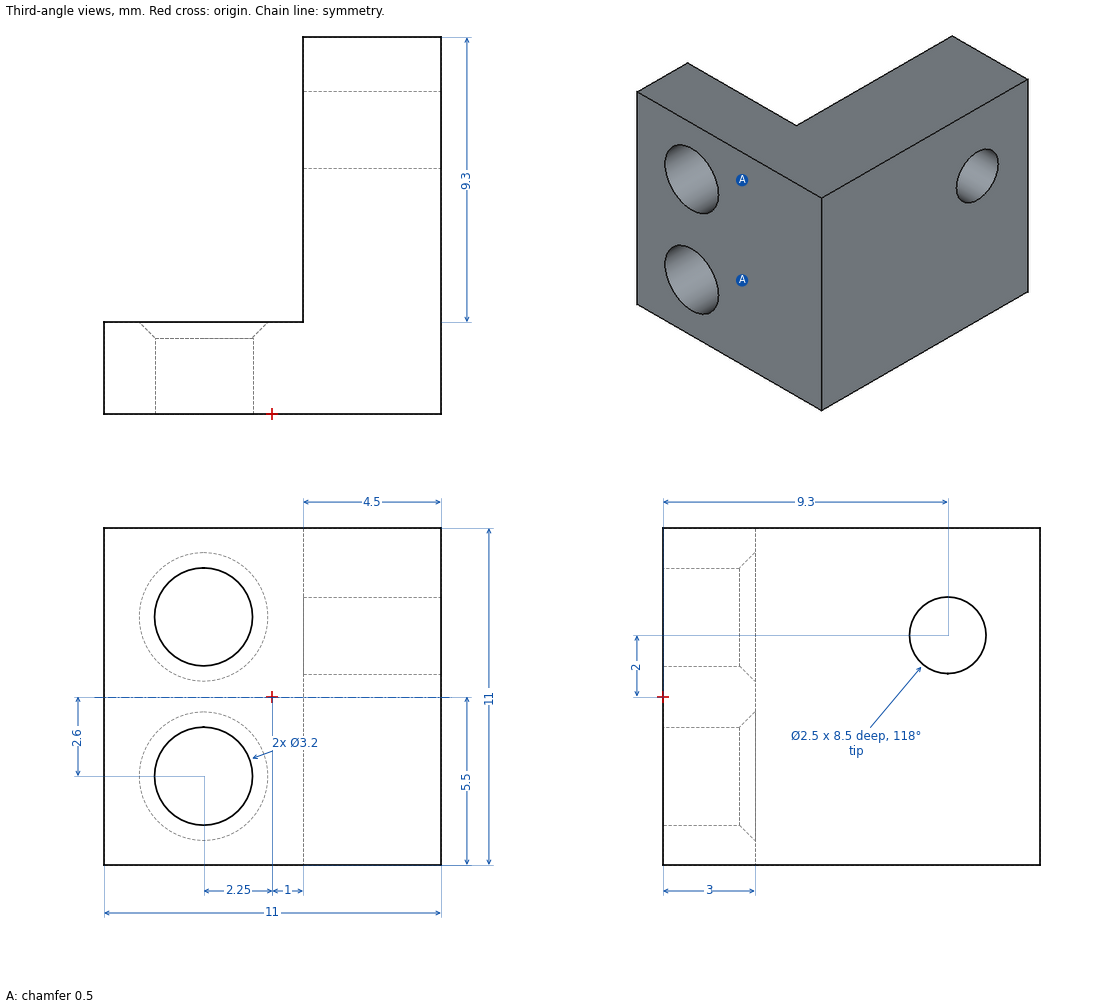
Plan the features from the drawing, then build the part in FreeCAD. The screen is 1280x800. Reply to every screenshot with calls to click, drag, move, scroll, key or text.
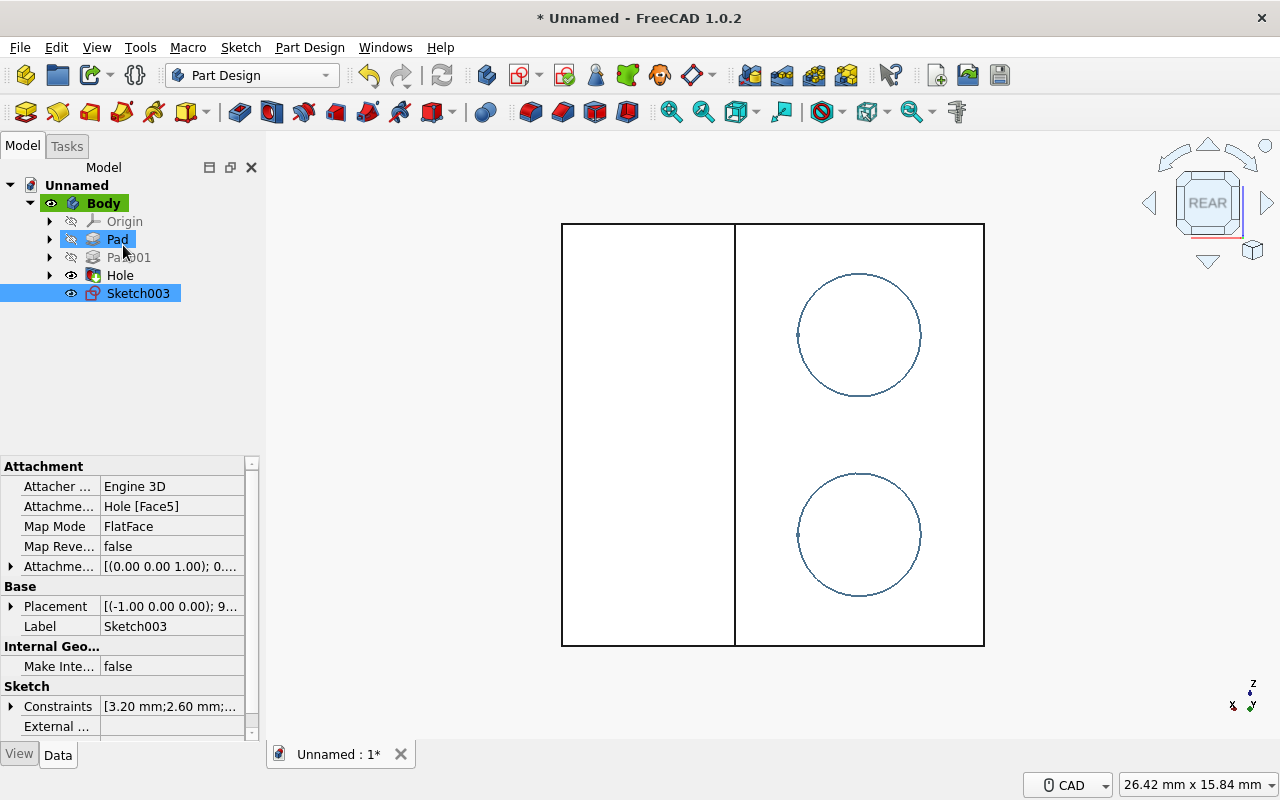
click(240, 112)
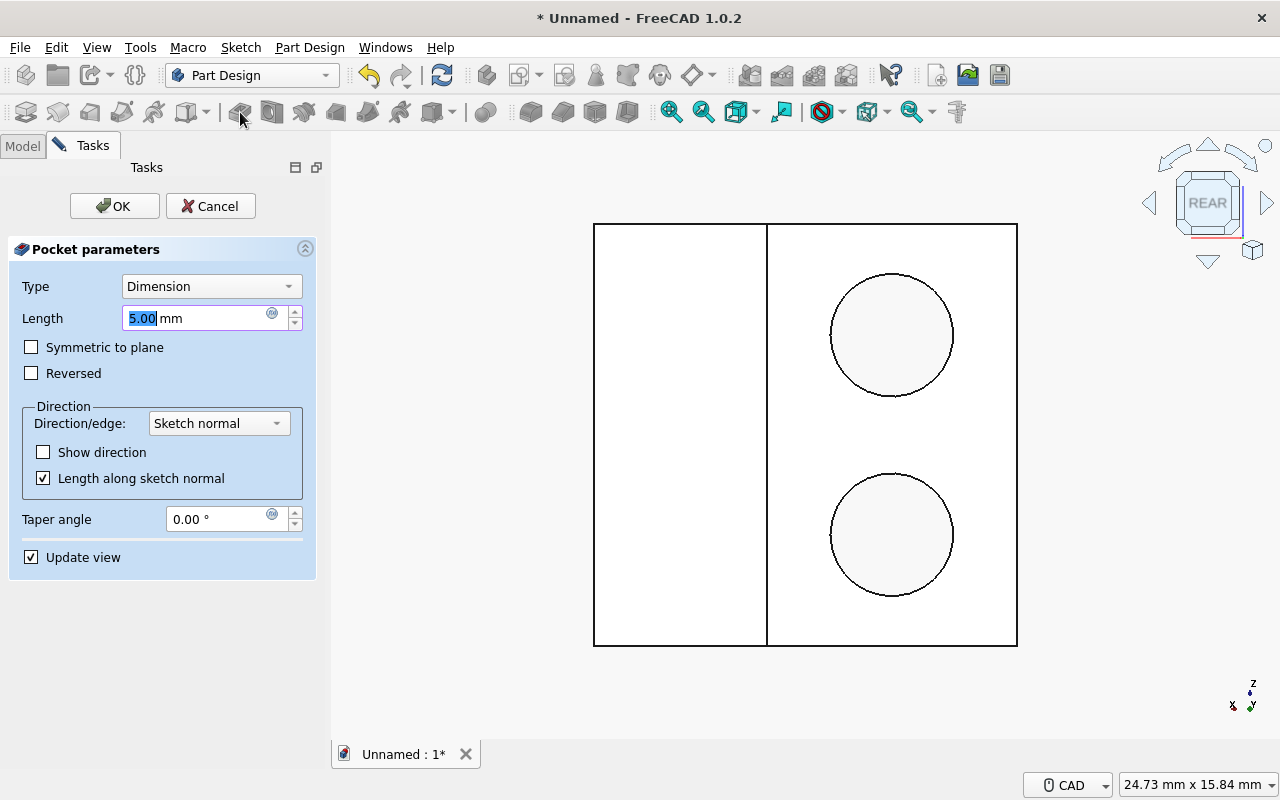
click(212, 286)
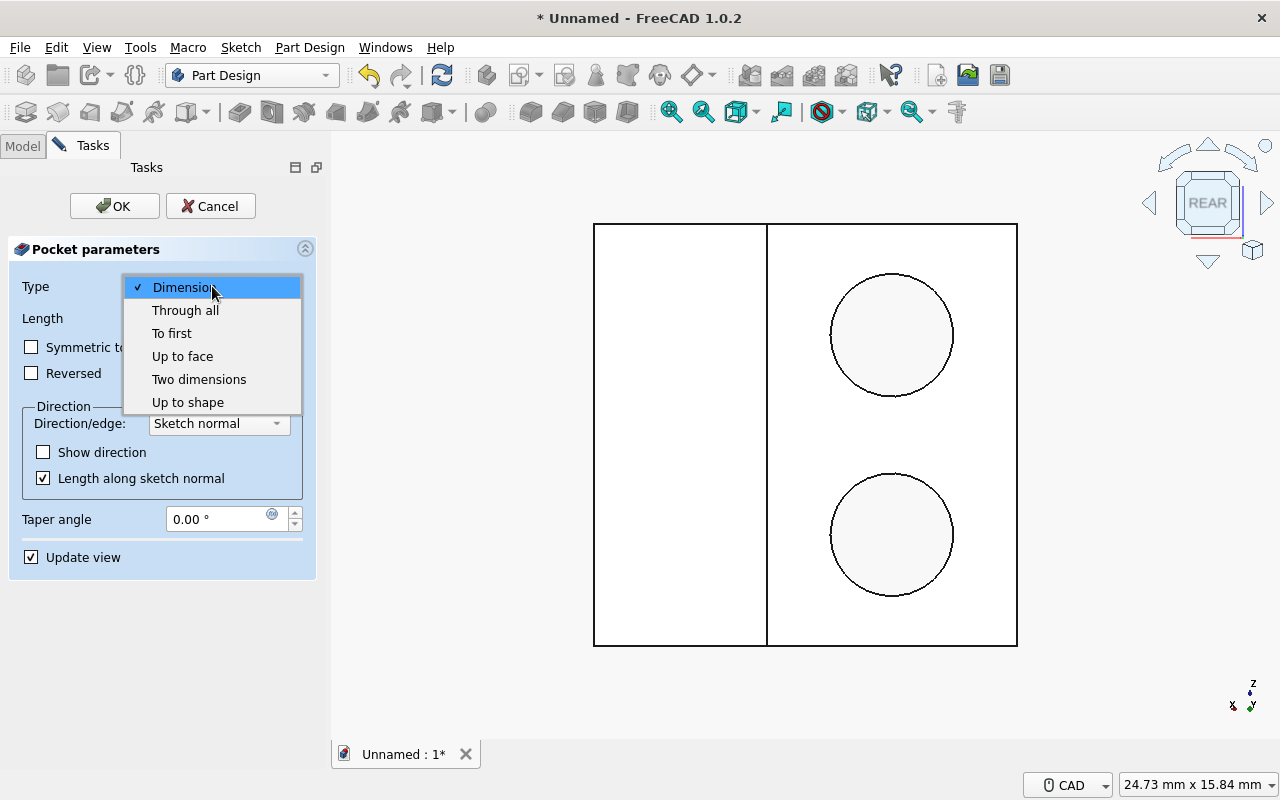
click(212, 310)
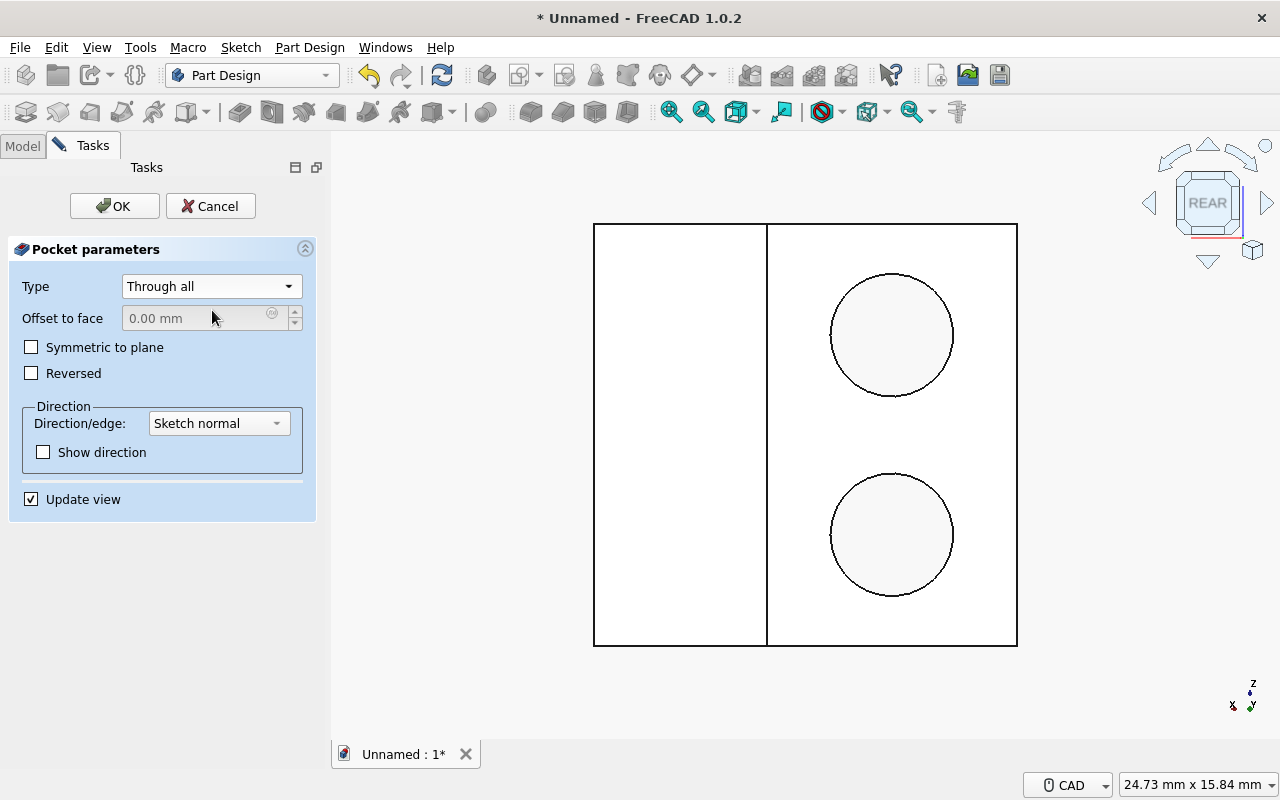
click(115, 206)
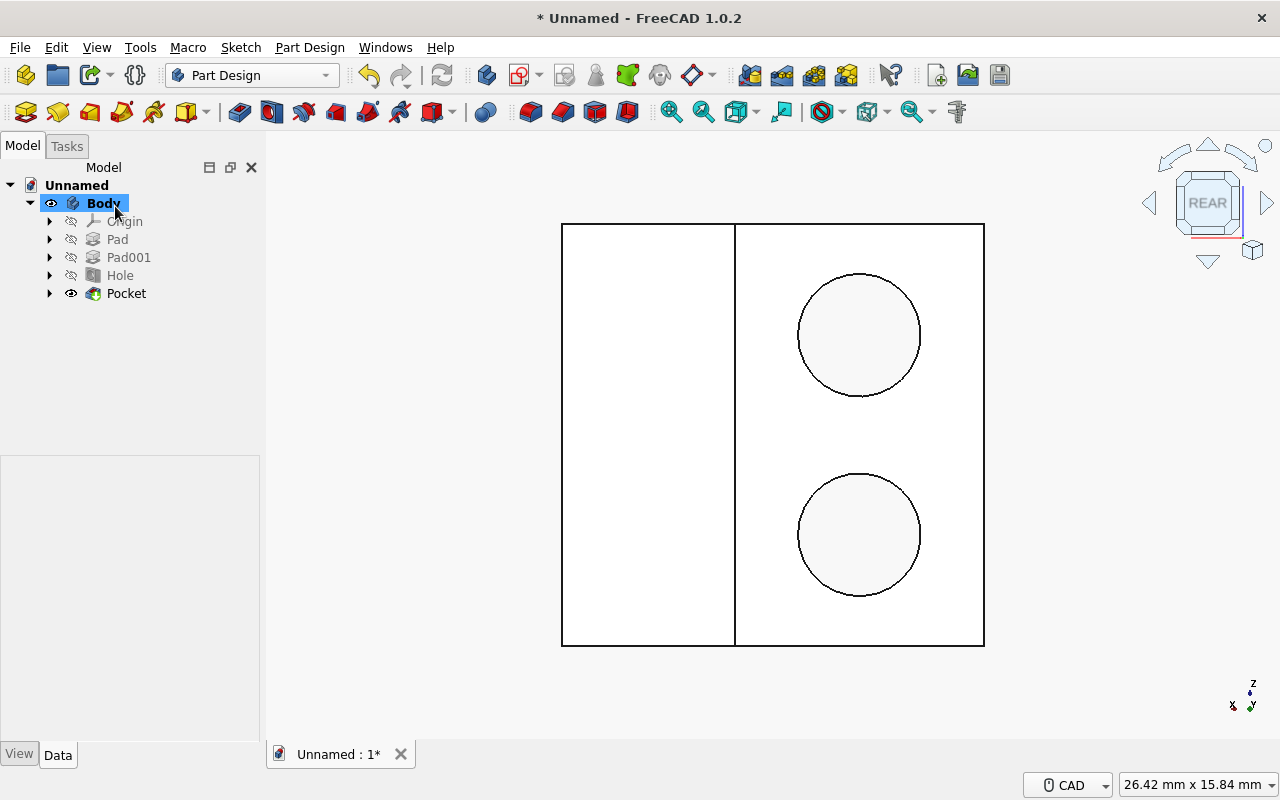
click(909, 498)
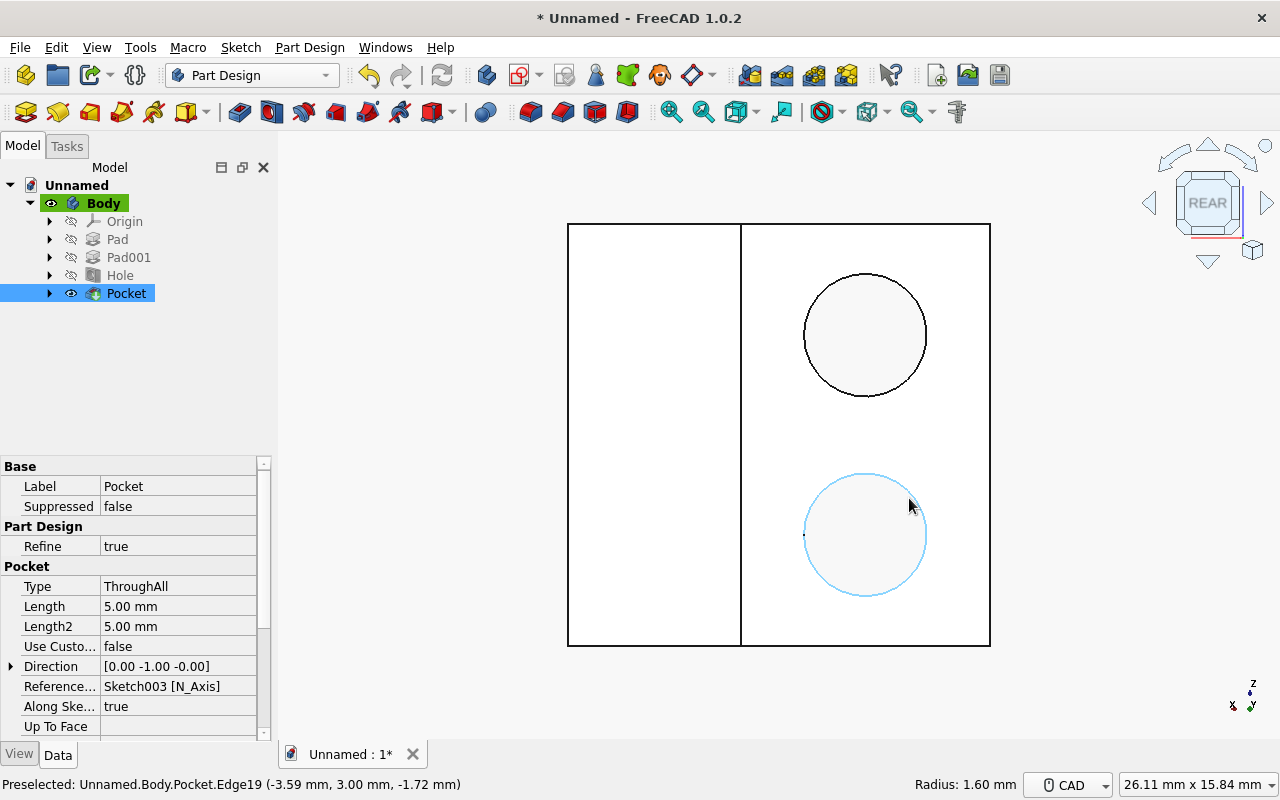
click(915, 298, ctrl)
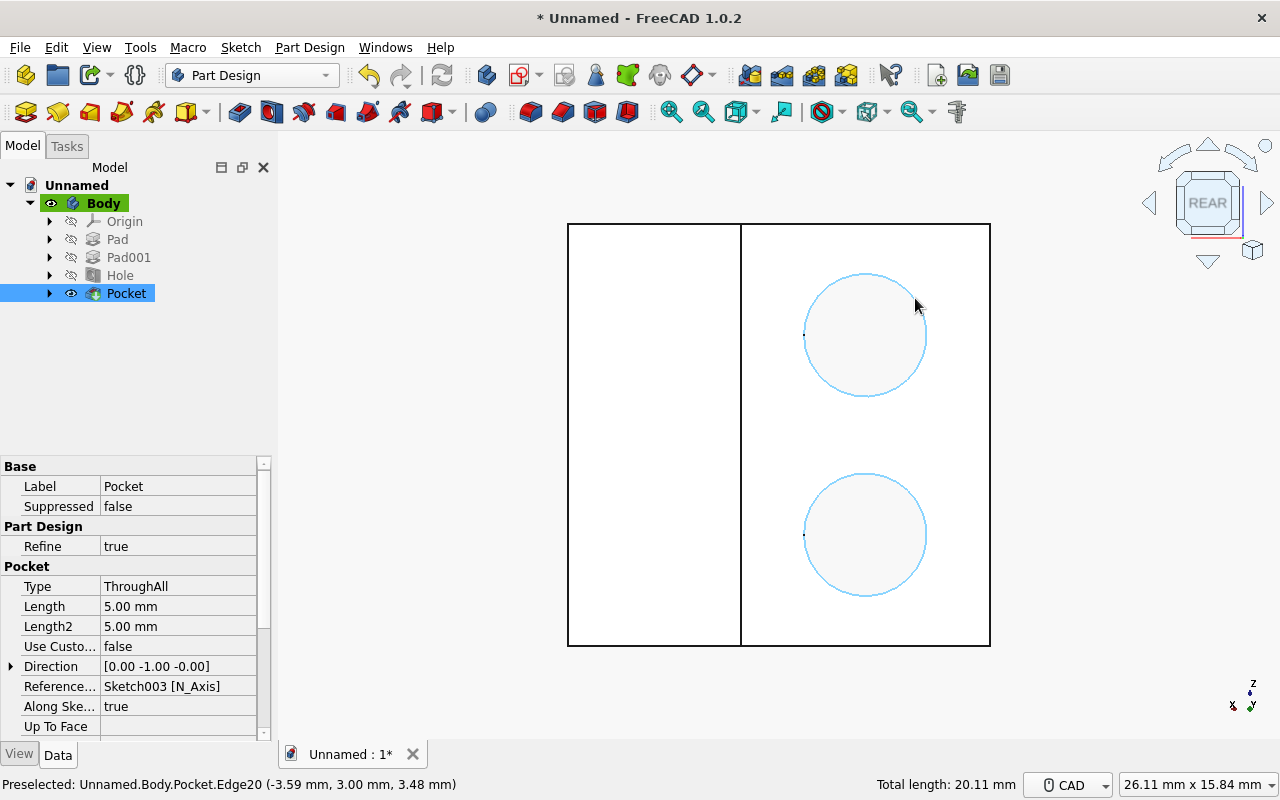
click(564, 112)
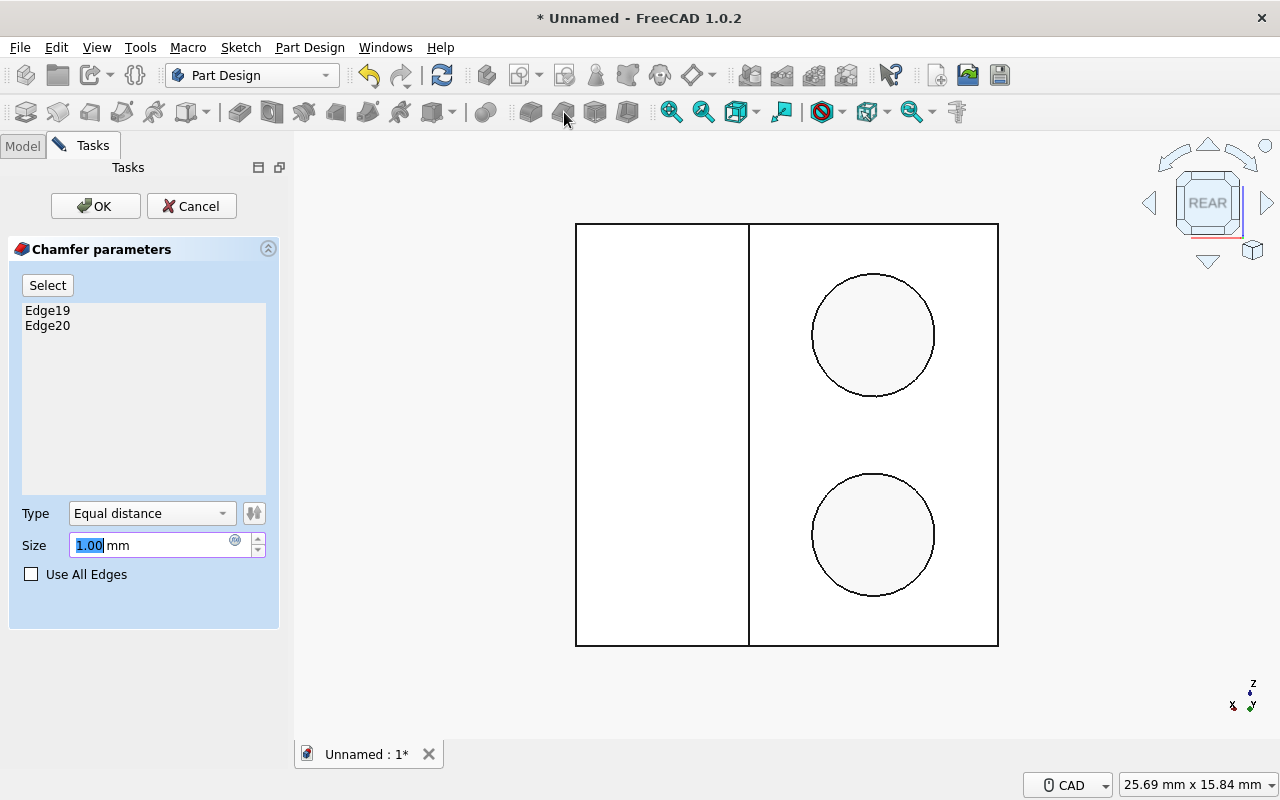
text(0.5)
key(Tab)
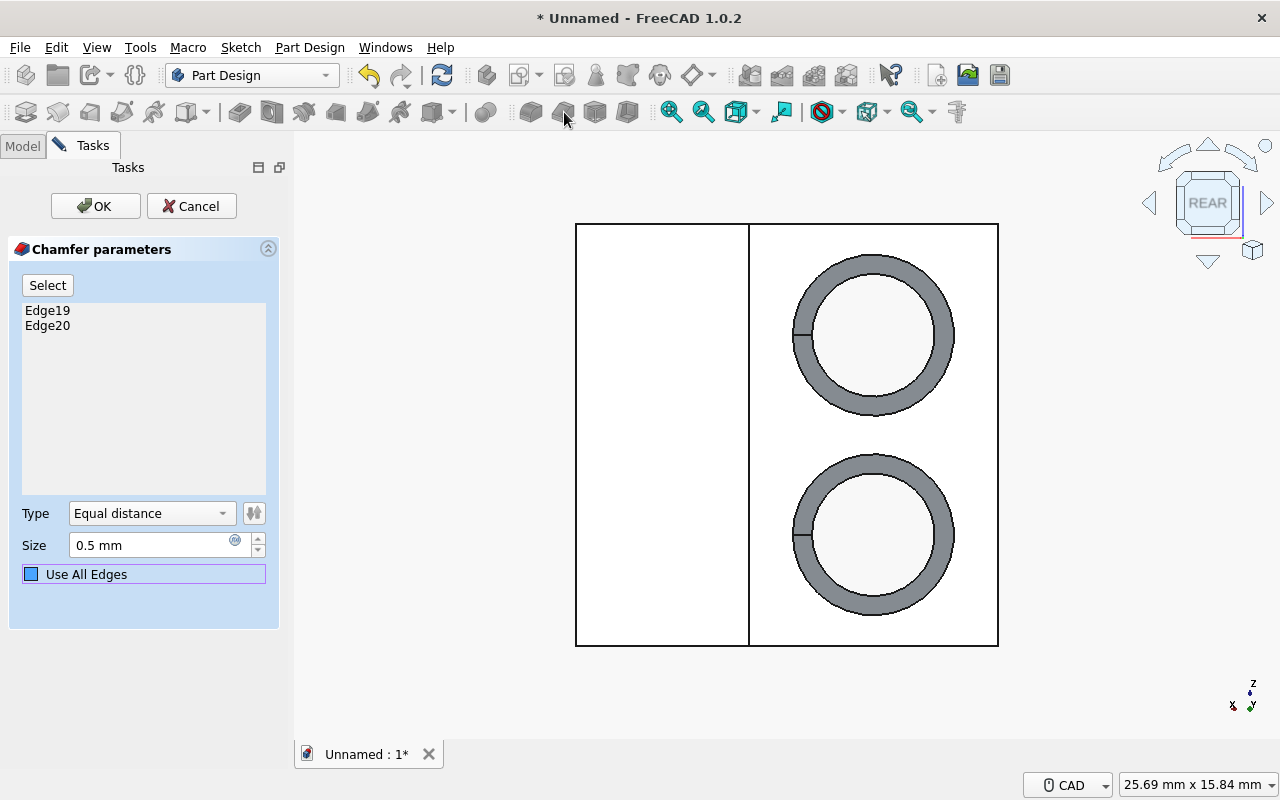
click(96, 206)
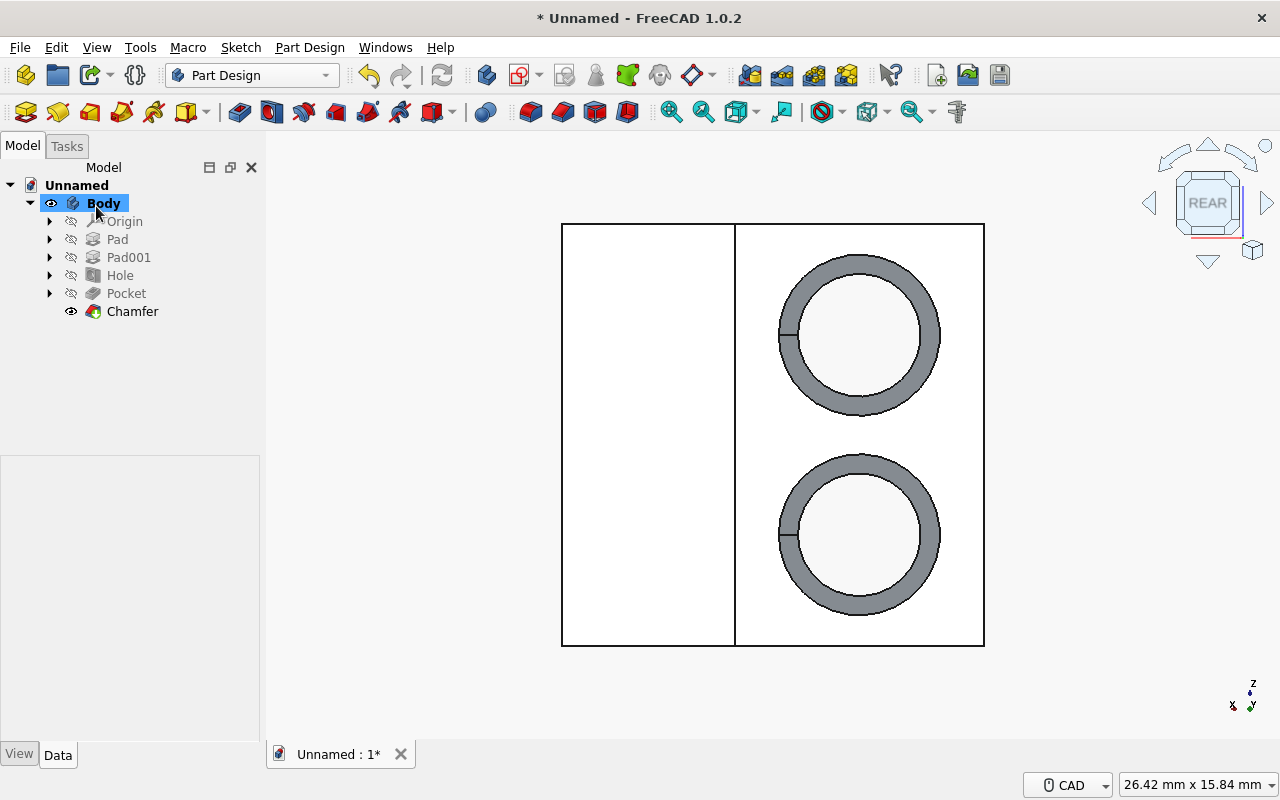
key(0)